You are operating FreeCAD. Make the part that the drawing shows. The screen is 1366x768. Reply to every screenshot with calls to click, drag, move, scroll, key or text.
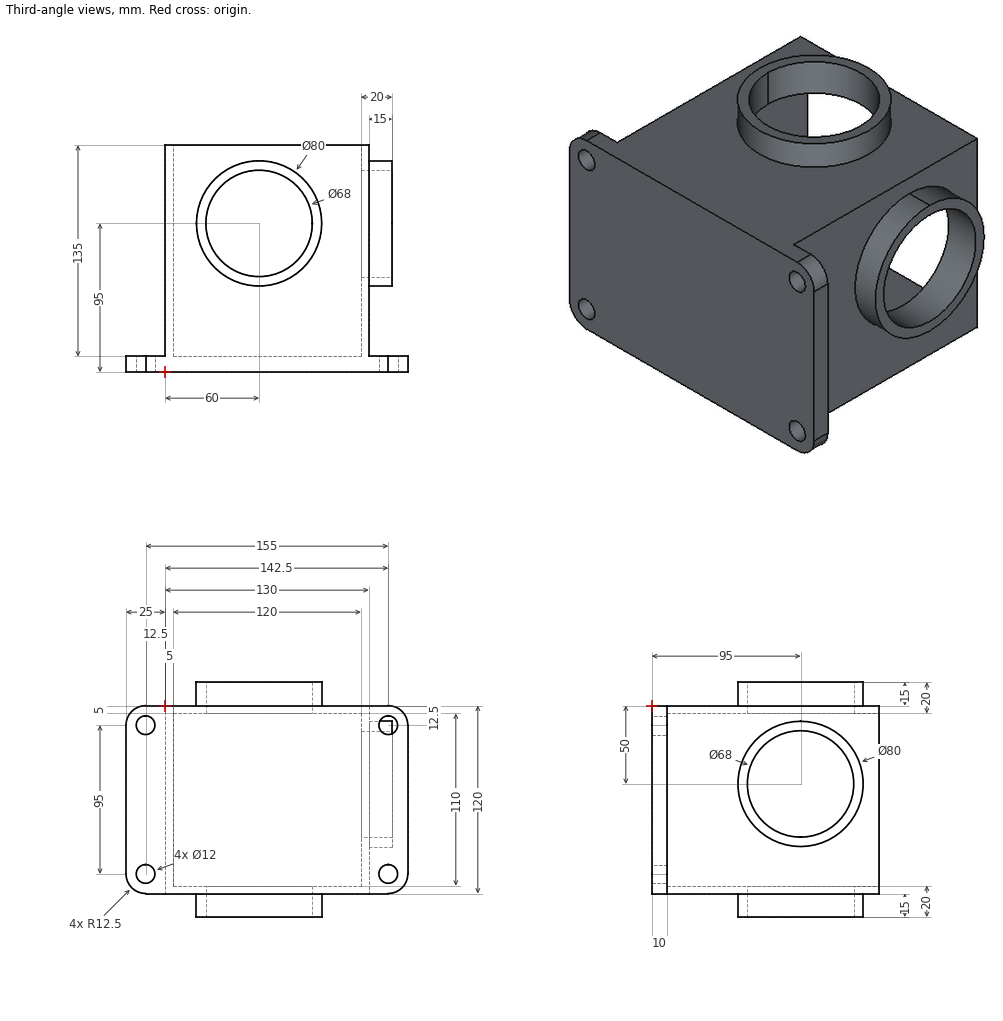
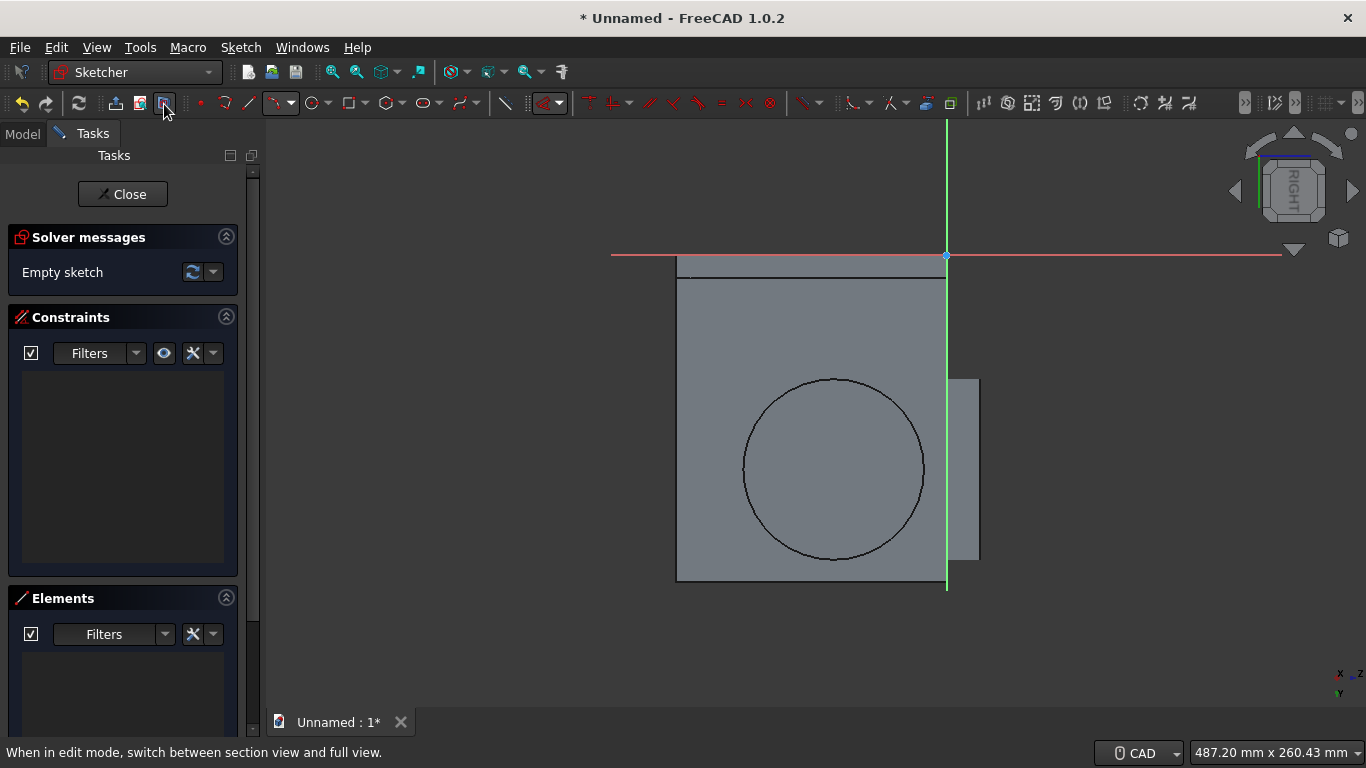
click(312, 104)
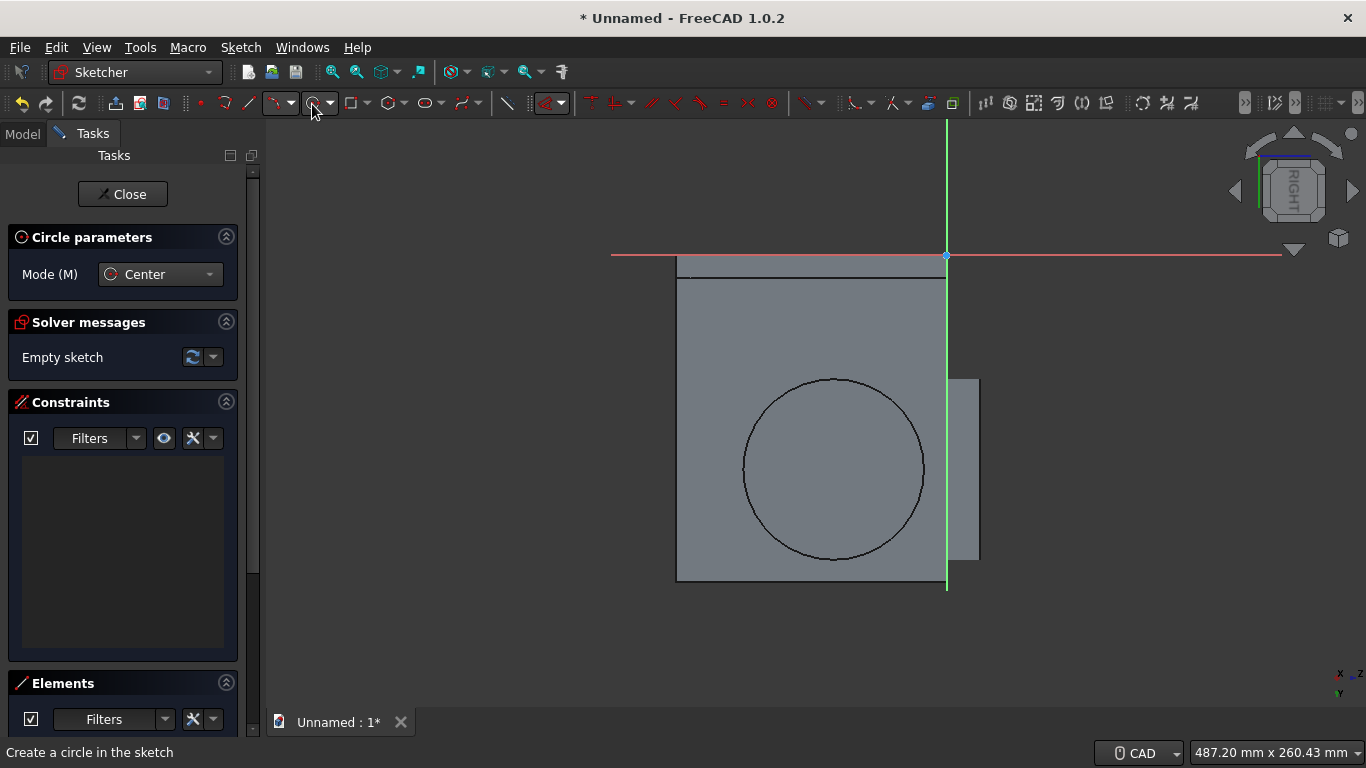
click(834, 470)
move(888, 415)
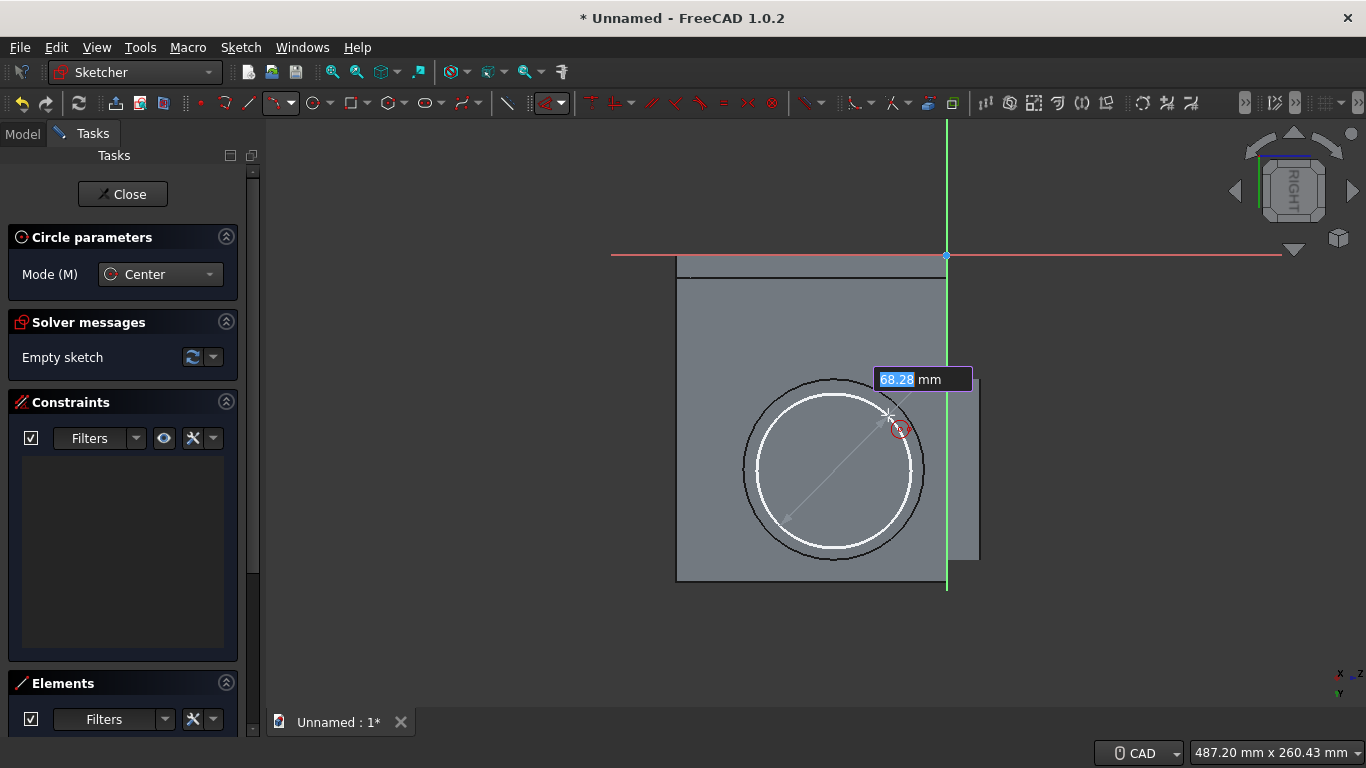
text(68)
key(Return)
key(Escape)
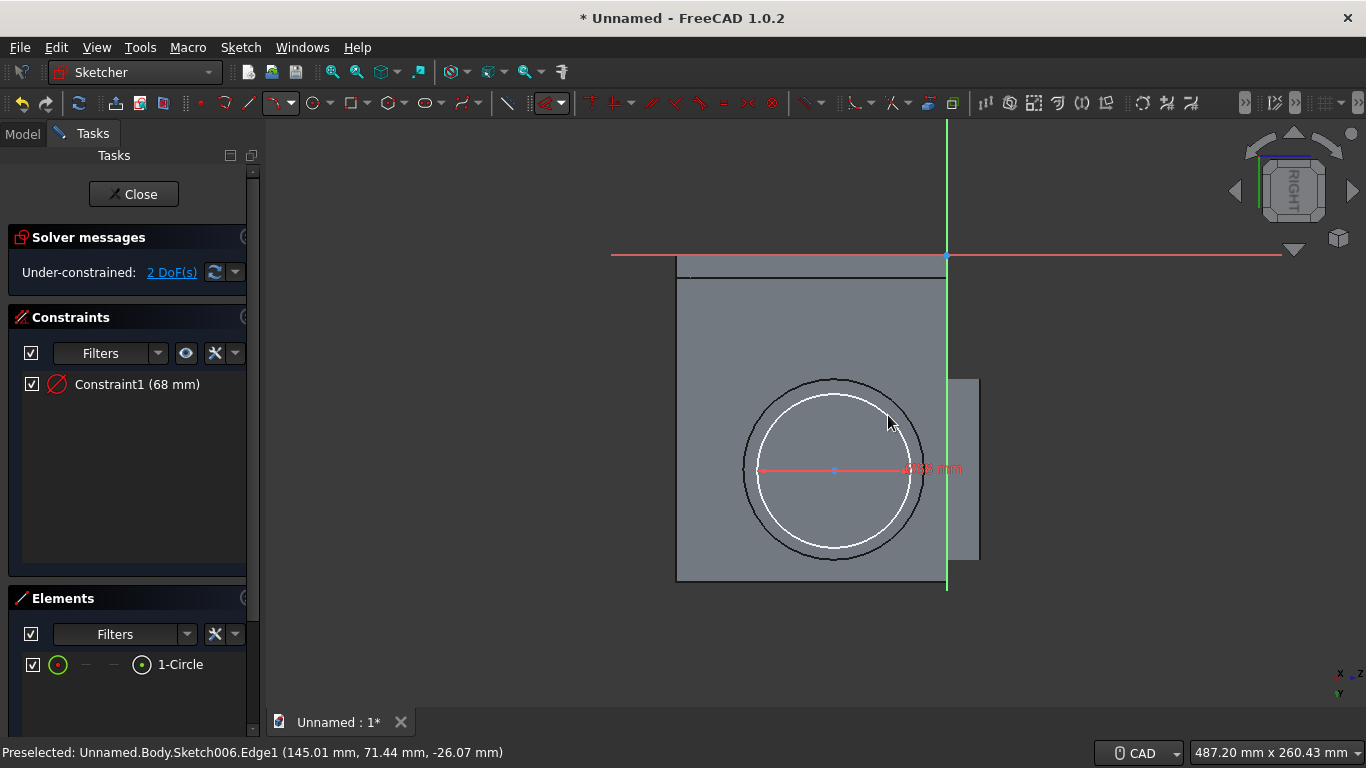
click(834, 471)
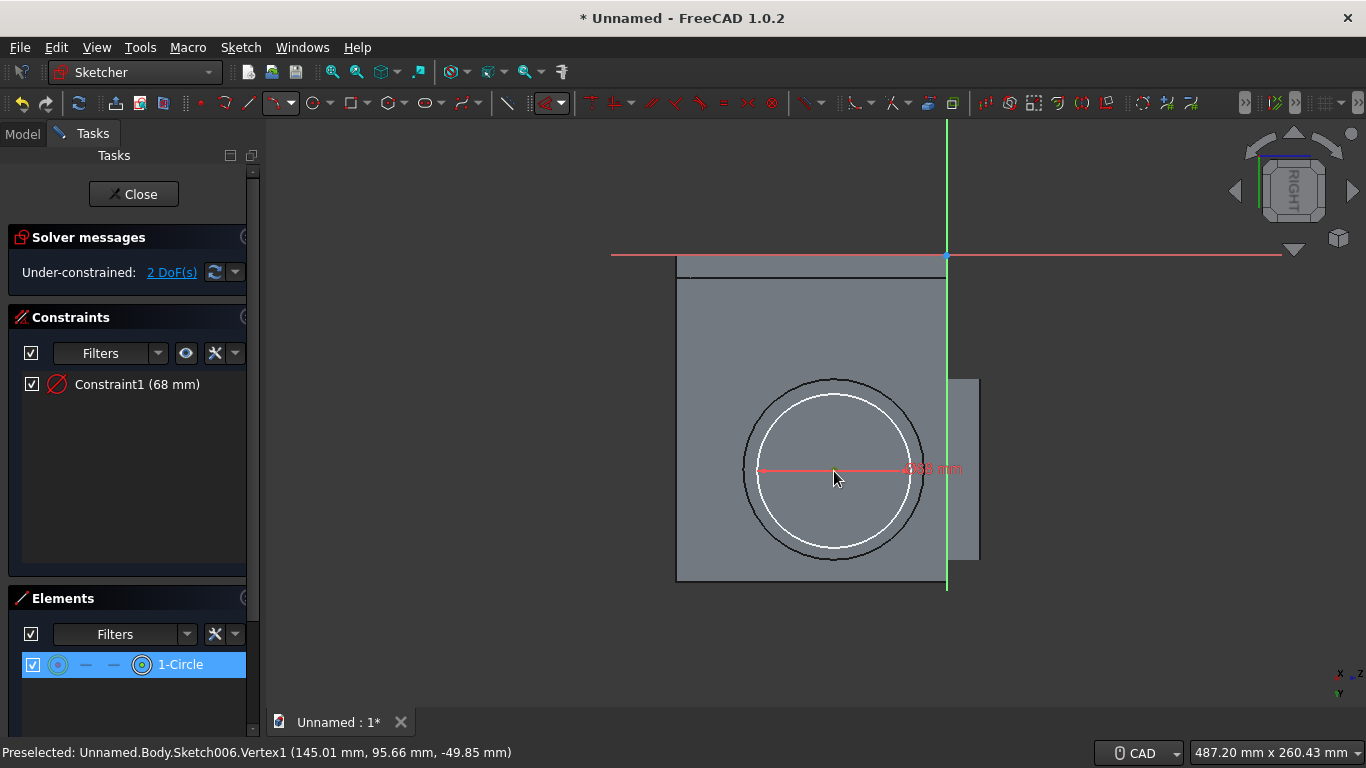
click(564, 104)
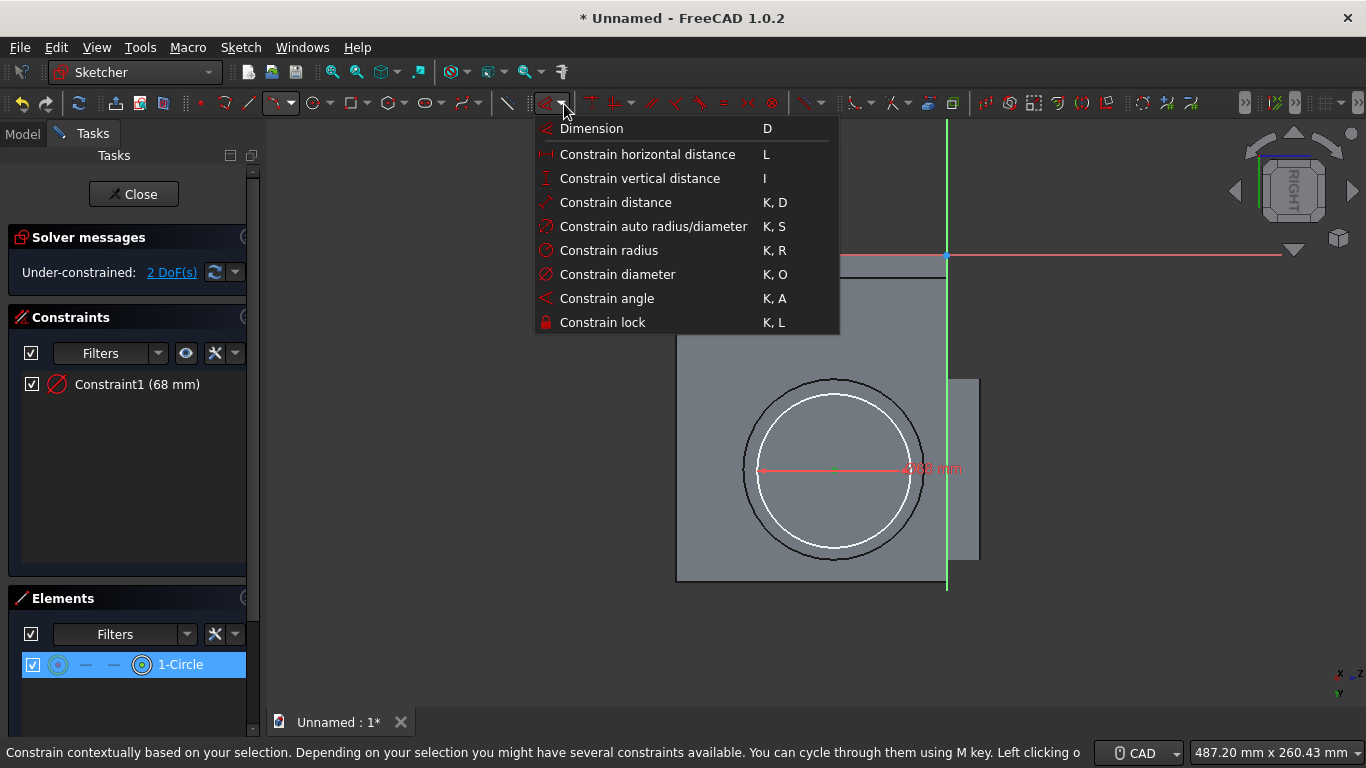
click(687, 154)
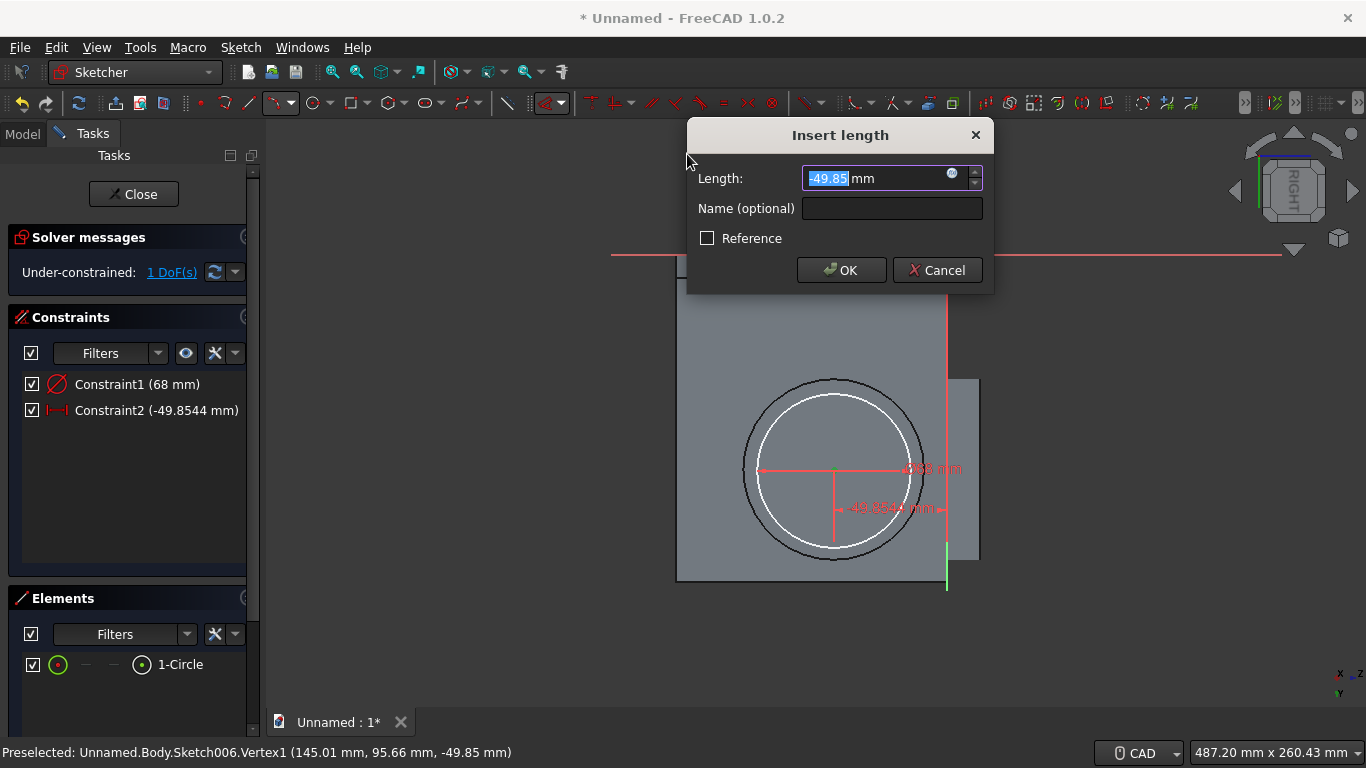
text(-50)
key(Return)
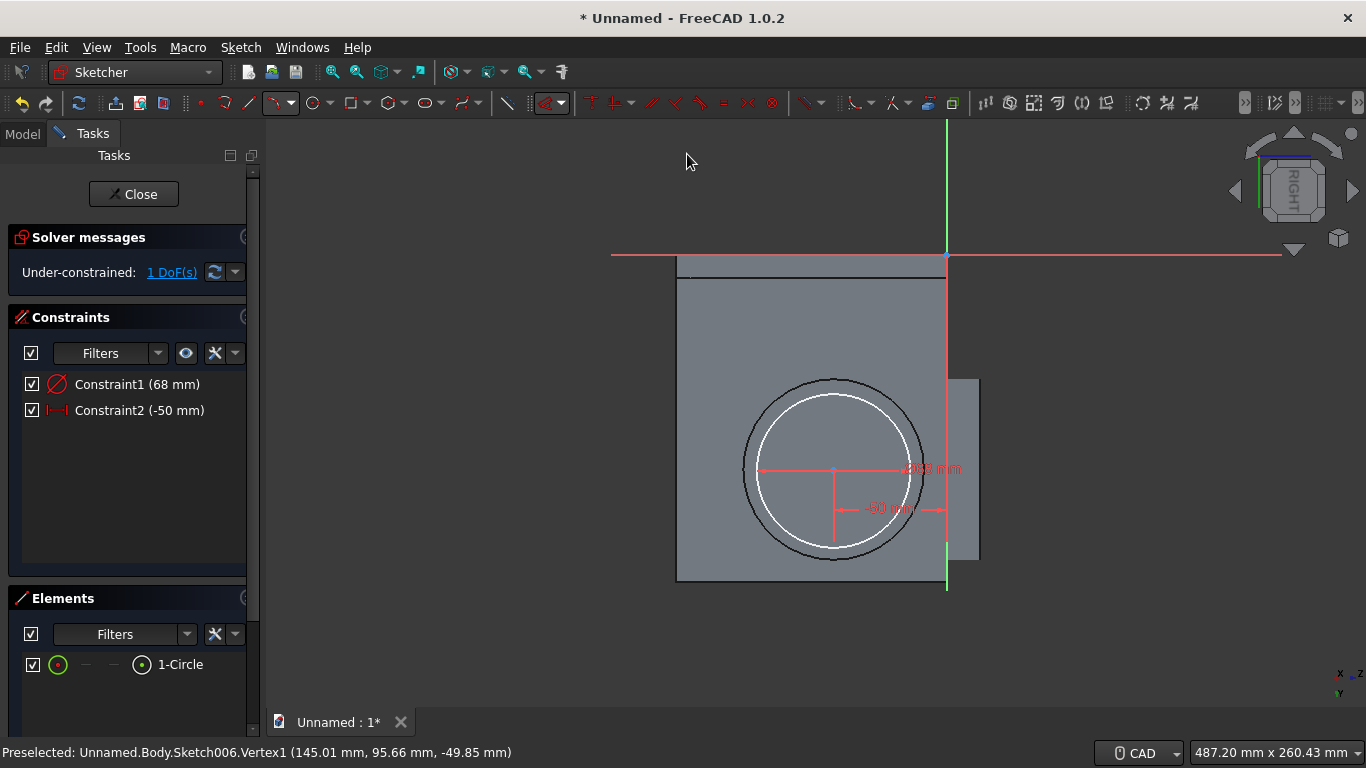
click(834, 471)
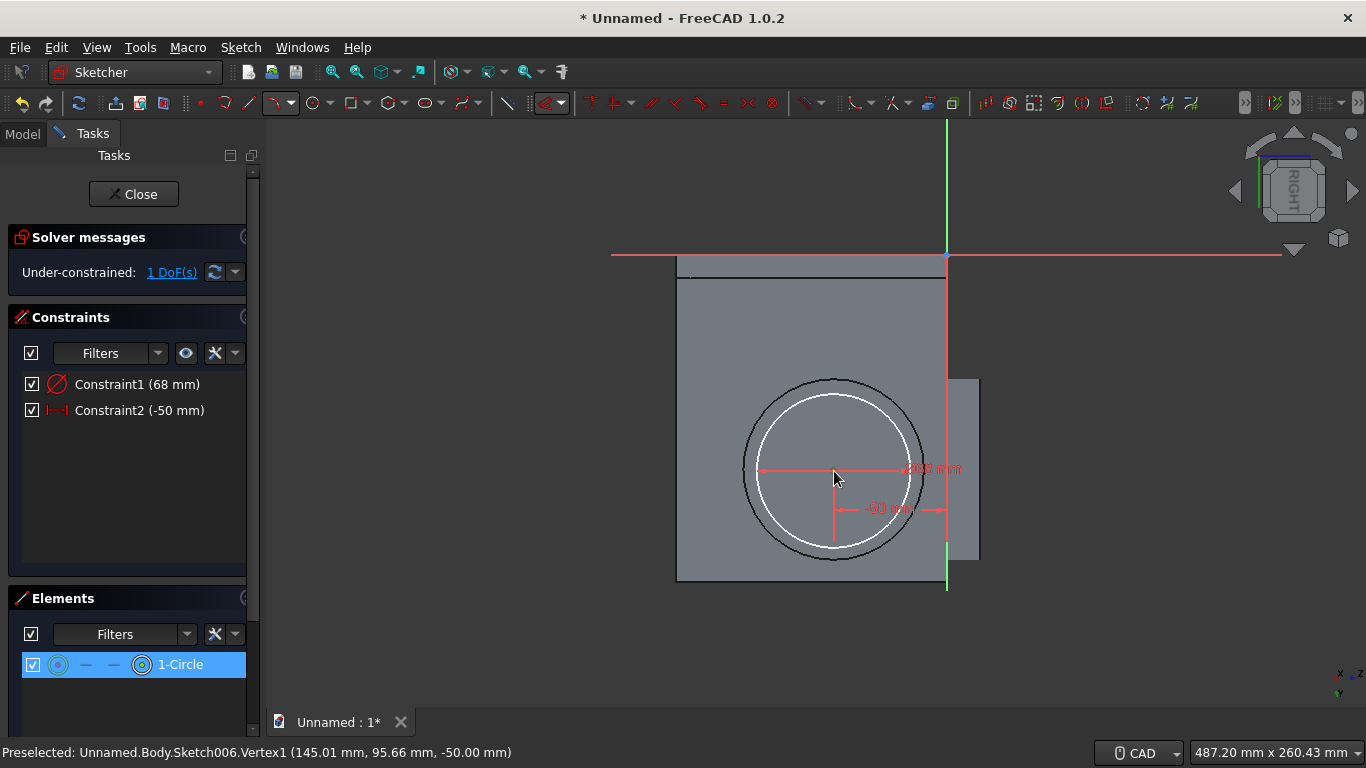
key(i)